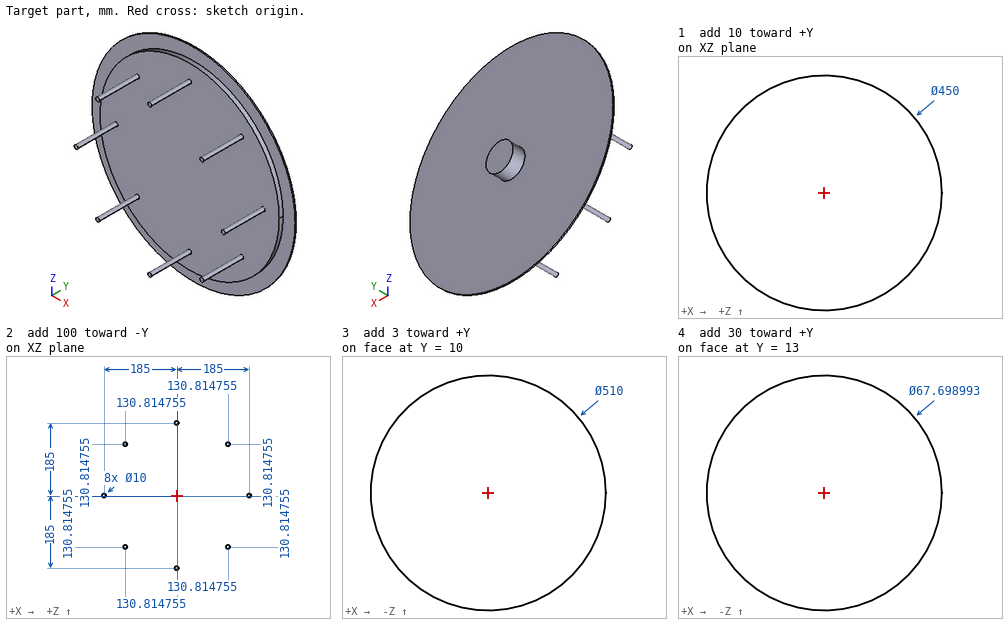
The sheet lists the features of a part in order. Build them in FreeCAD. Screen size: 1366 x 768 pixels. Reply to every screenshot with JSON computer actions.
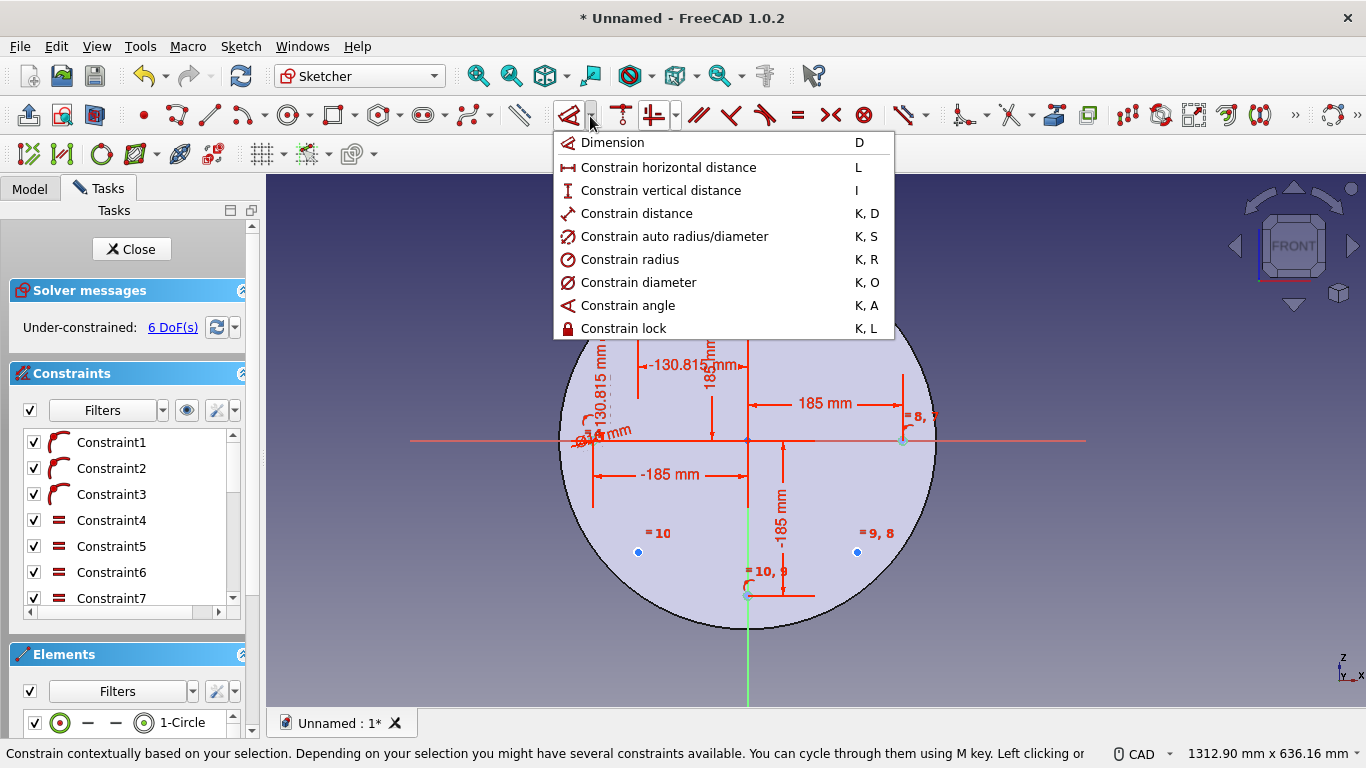
{"action": "left_click", "coordinate": [724, 168]}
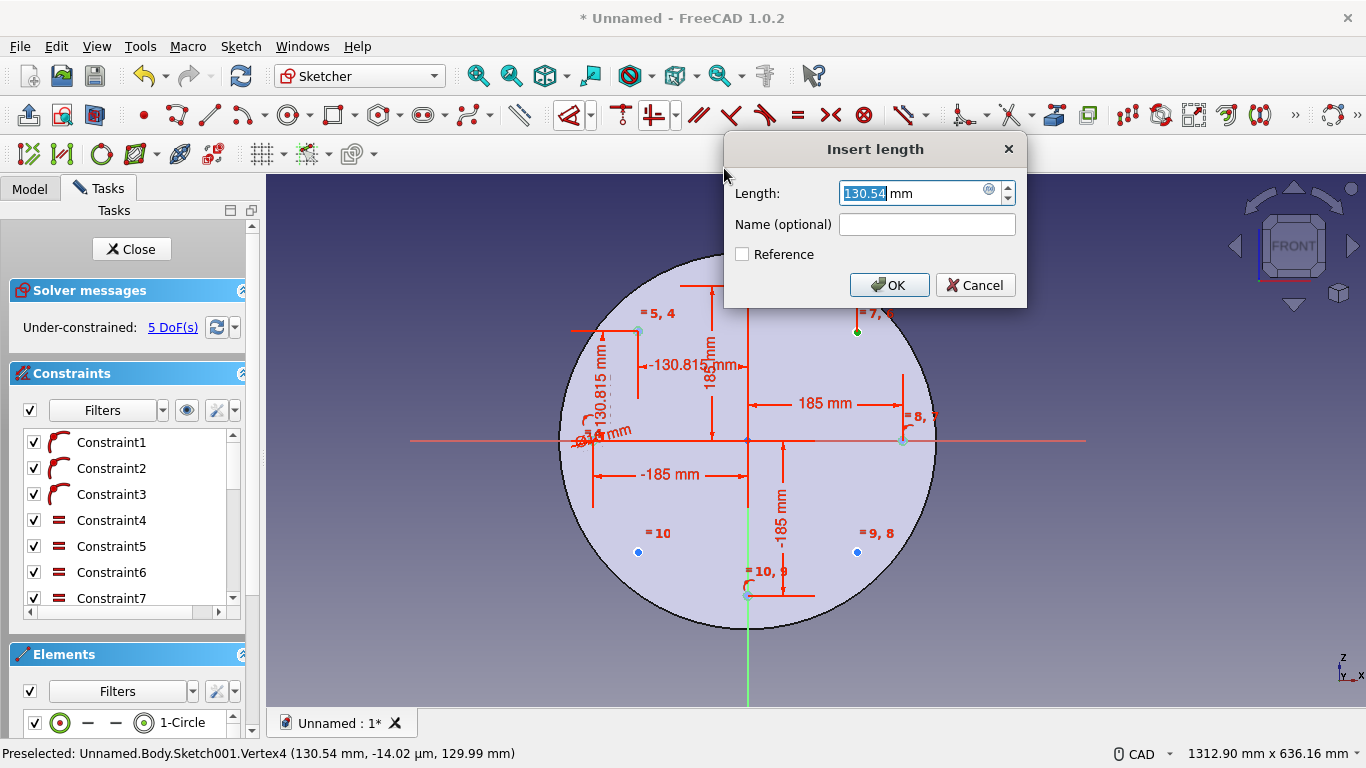
{"action": "type", "text": "130.814755"}
{"action": "key", "text": "Return"}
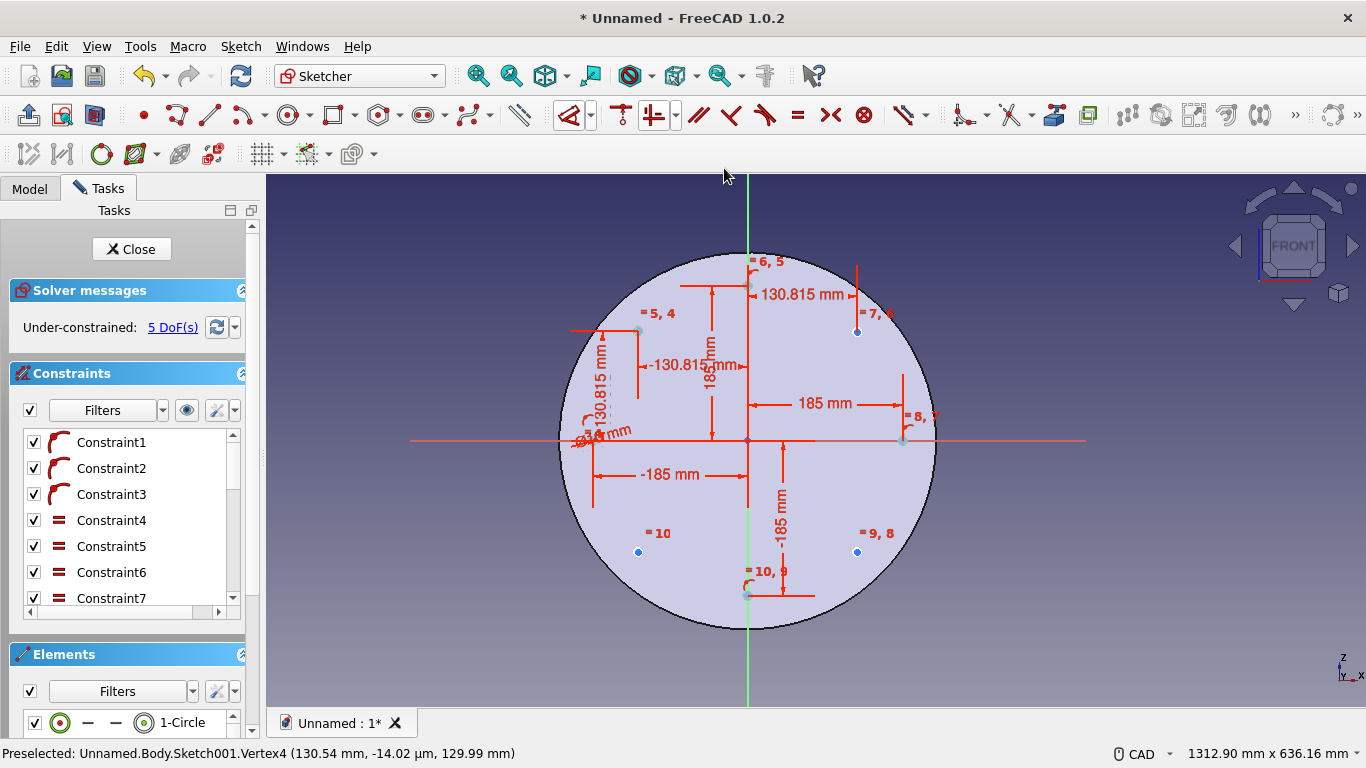
{"action": "left_click", "coordinate": [857, 332]}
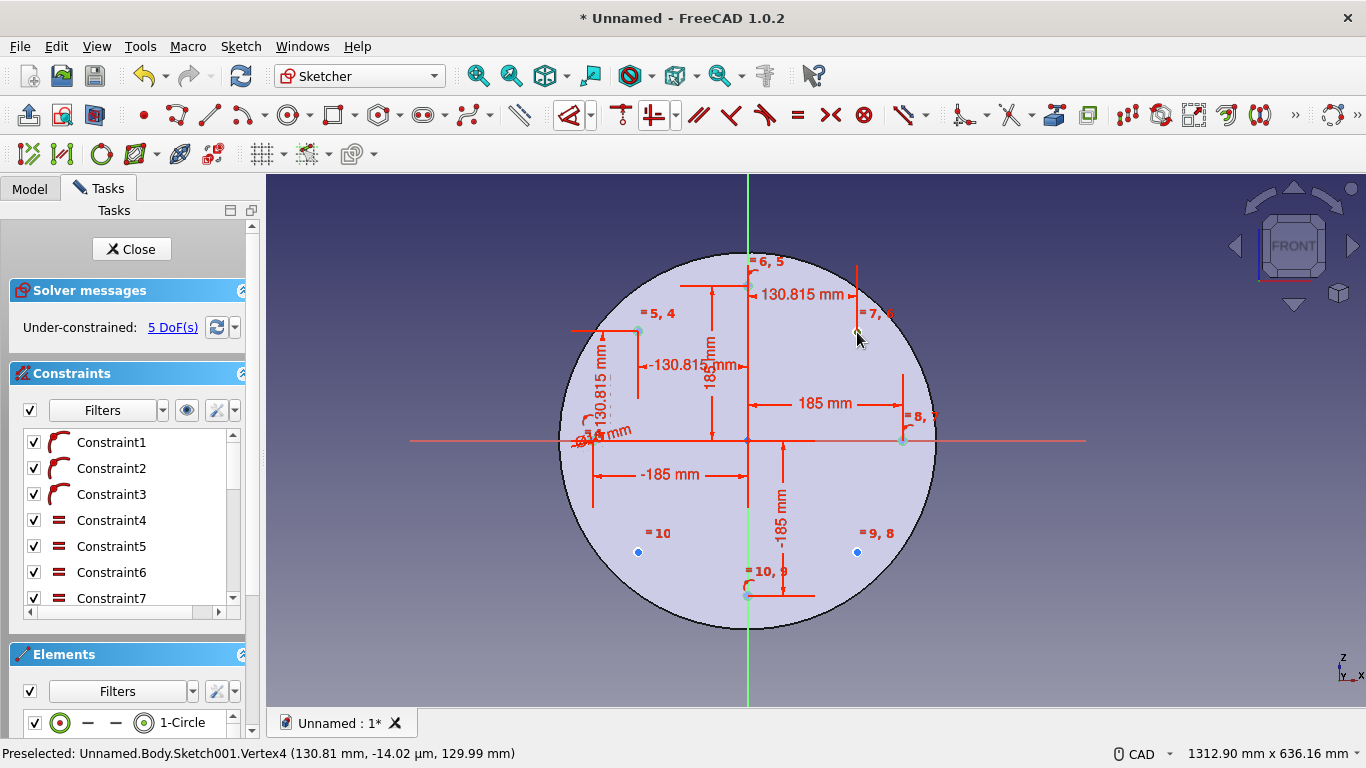
{"action": "left_click", "coordinate": [590, 116]}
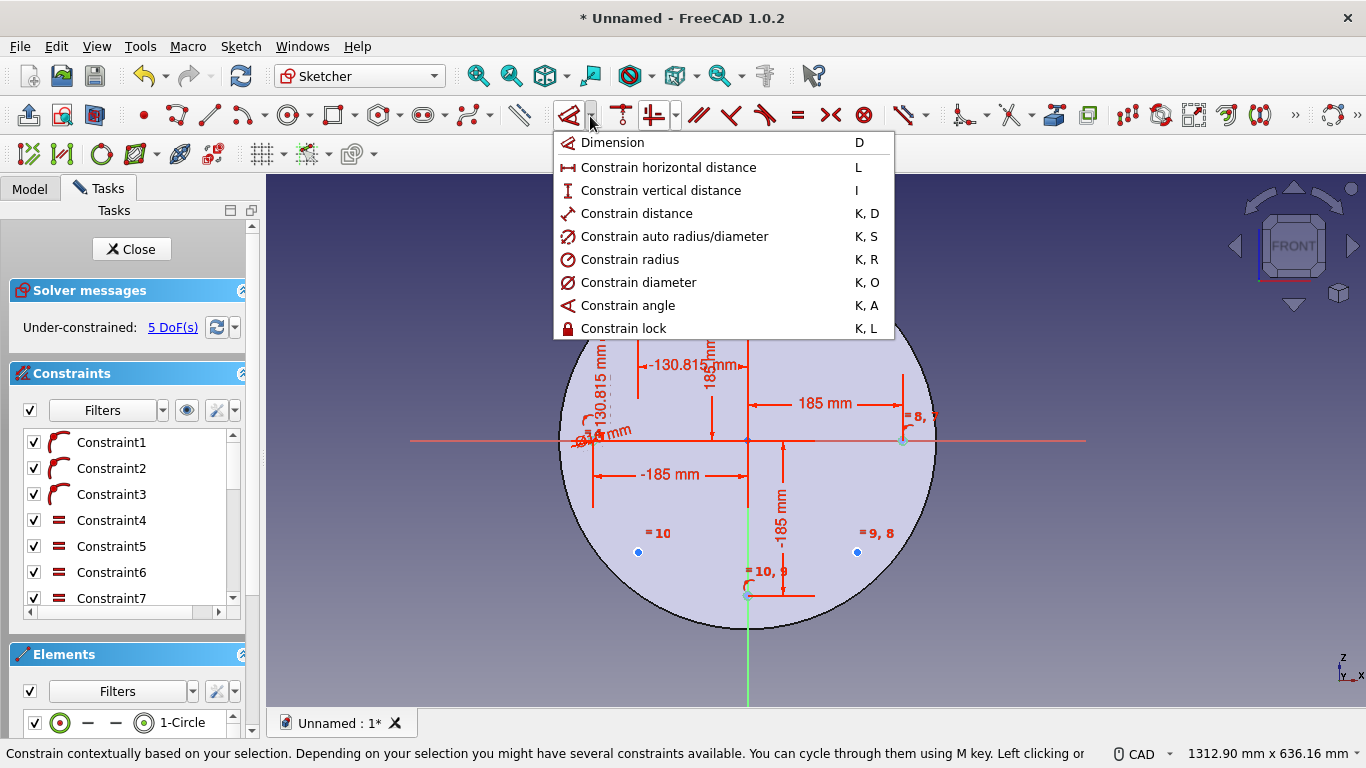
{"action": "left_click", "coordinate": [724, 190]}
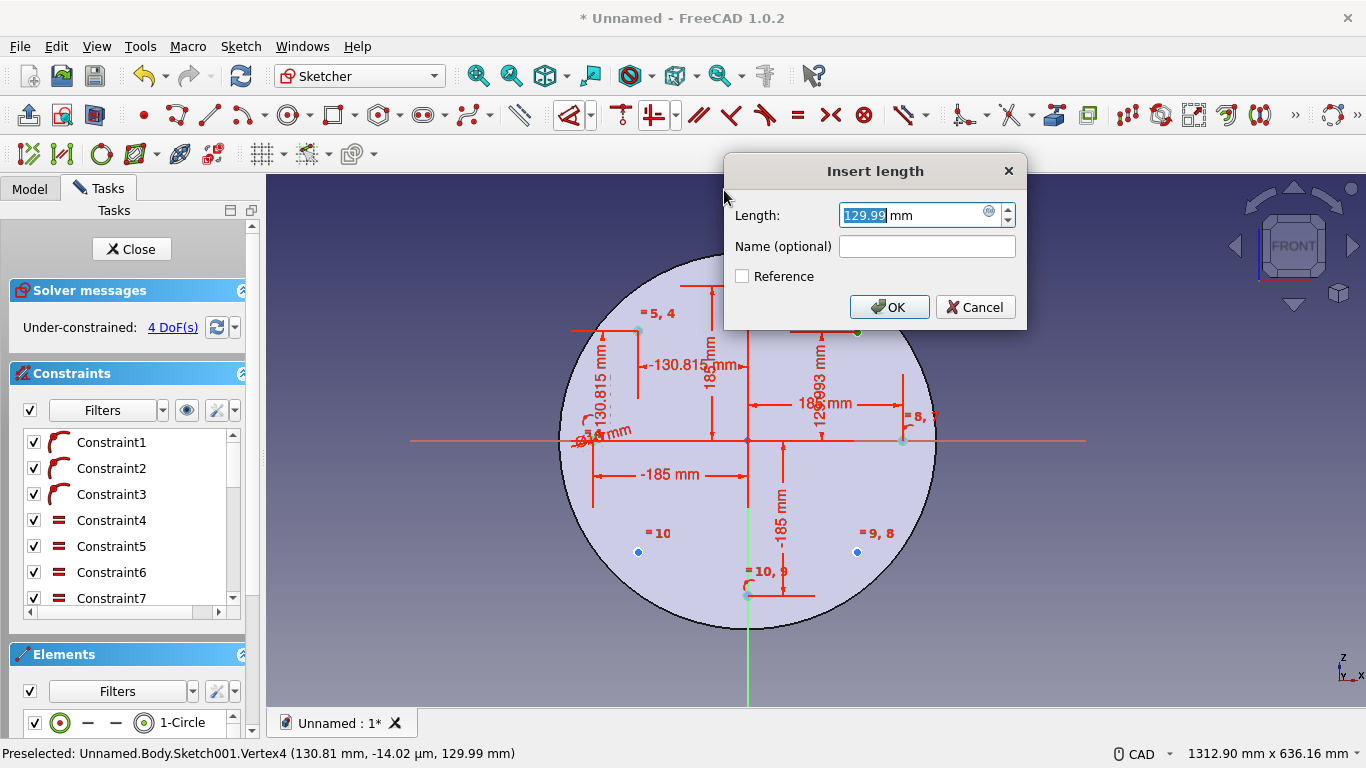
{"action": "type", "text": "130.814755"}
{"action": "key", "text": "Return"}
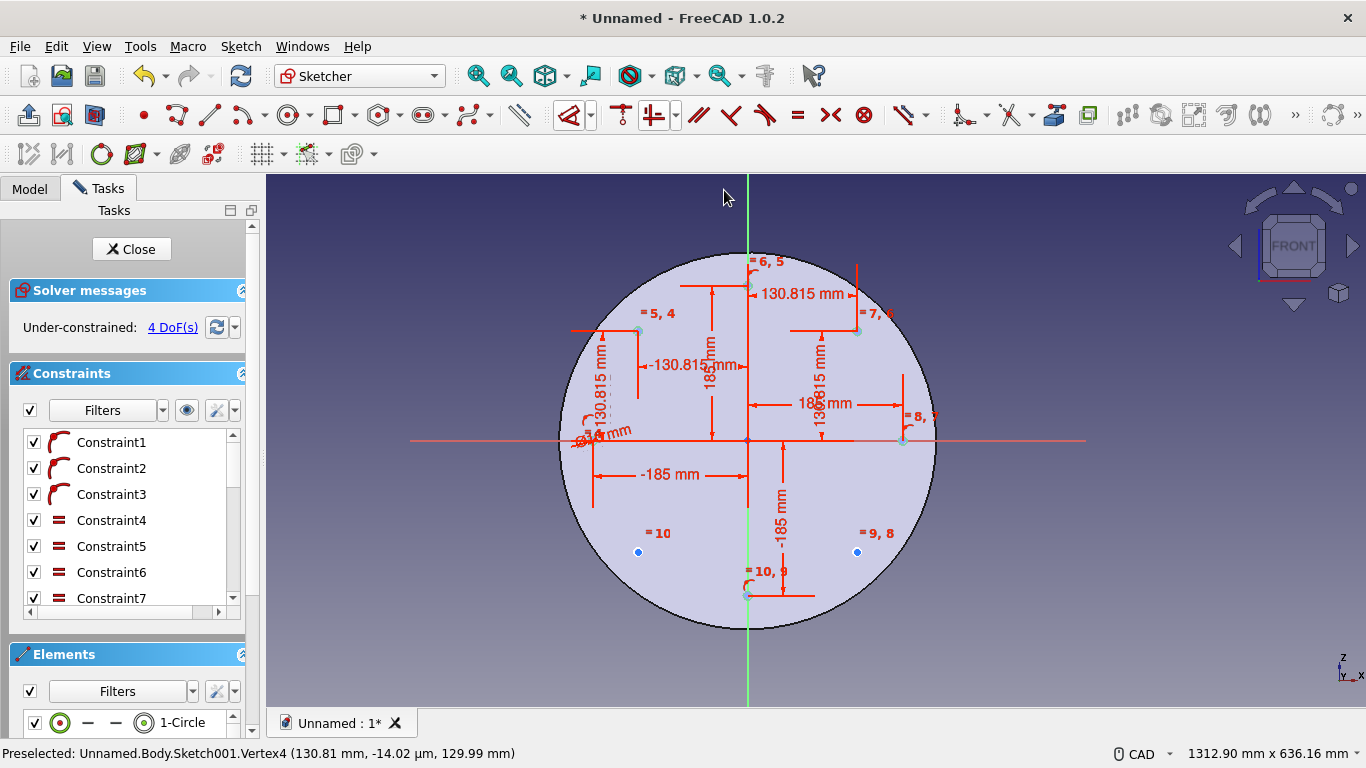
{"action": "left_click", "coordinate": [857, 552]}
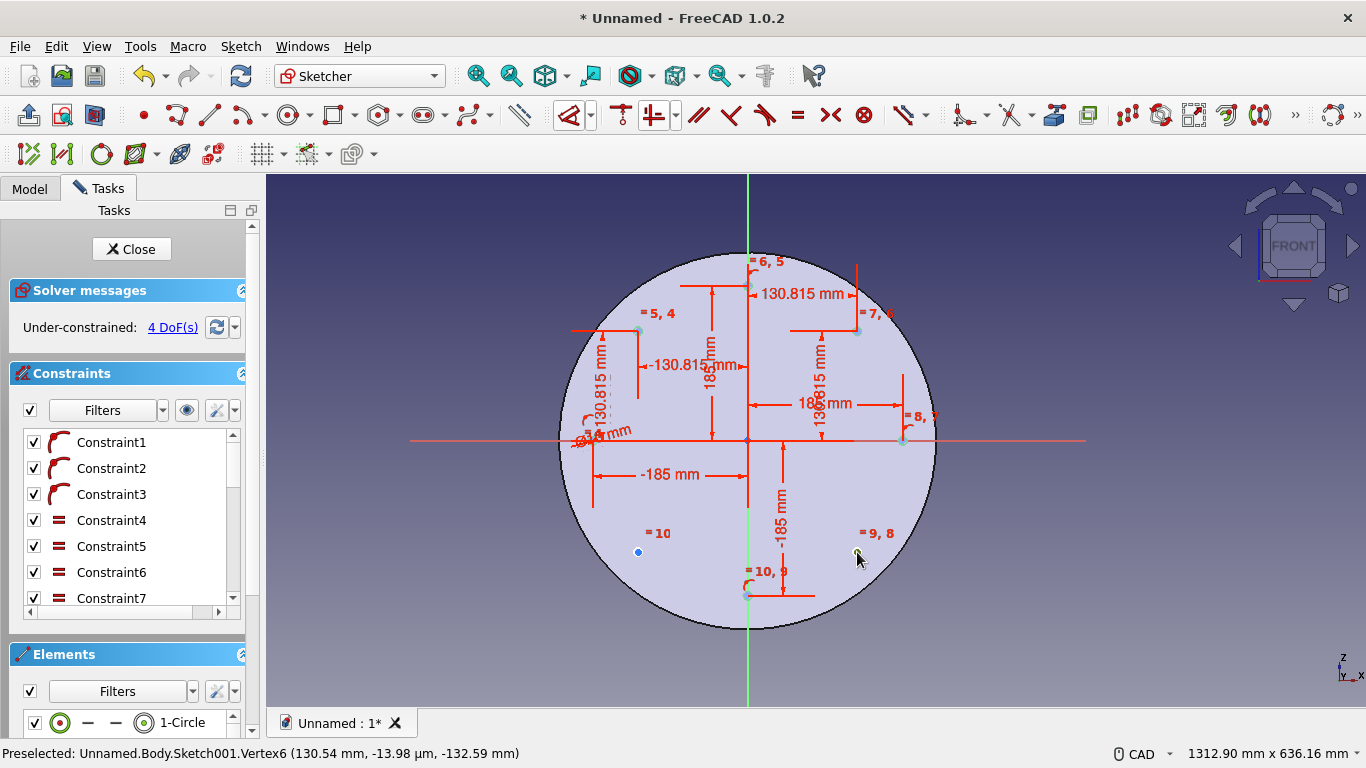
{"action": "left_click", "coordinate": [590, 116]}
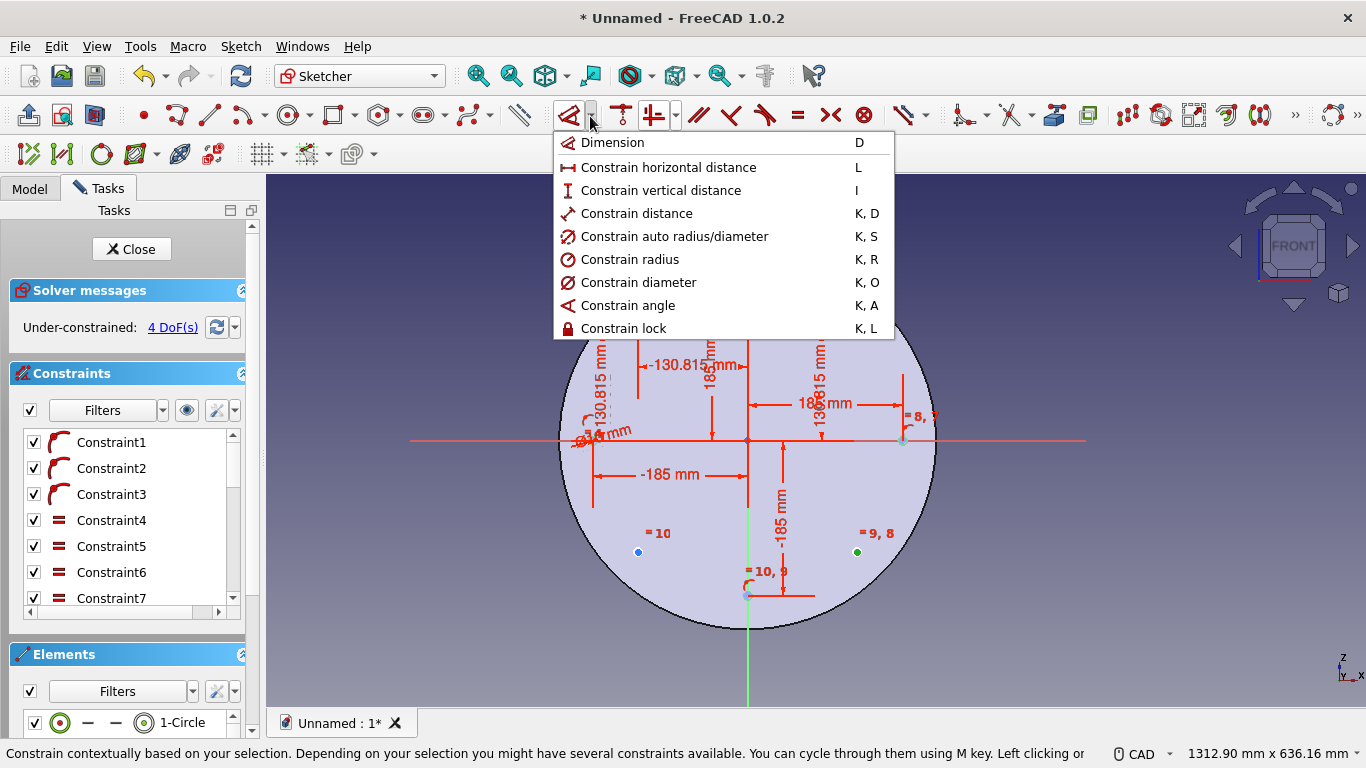
{"action": "left_click", "coordinate": [724, 168]}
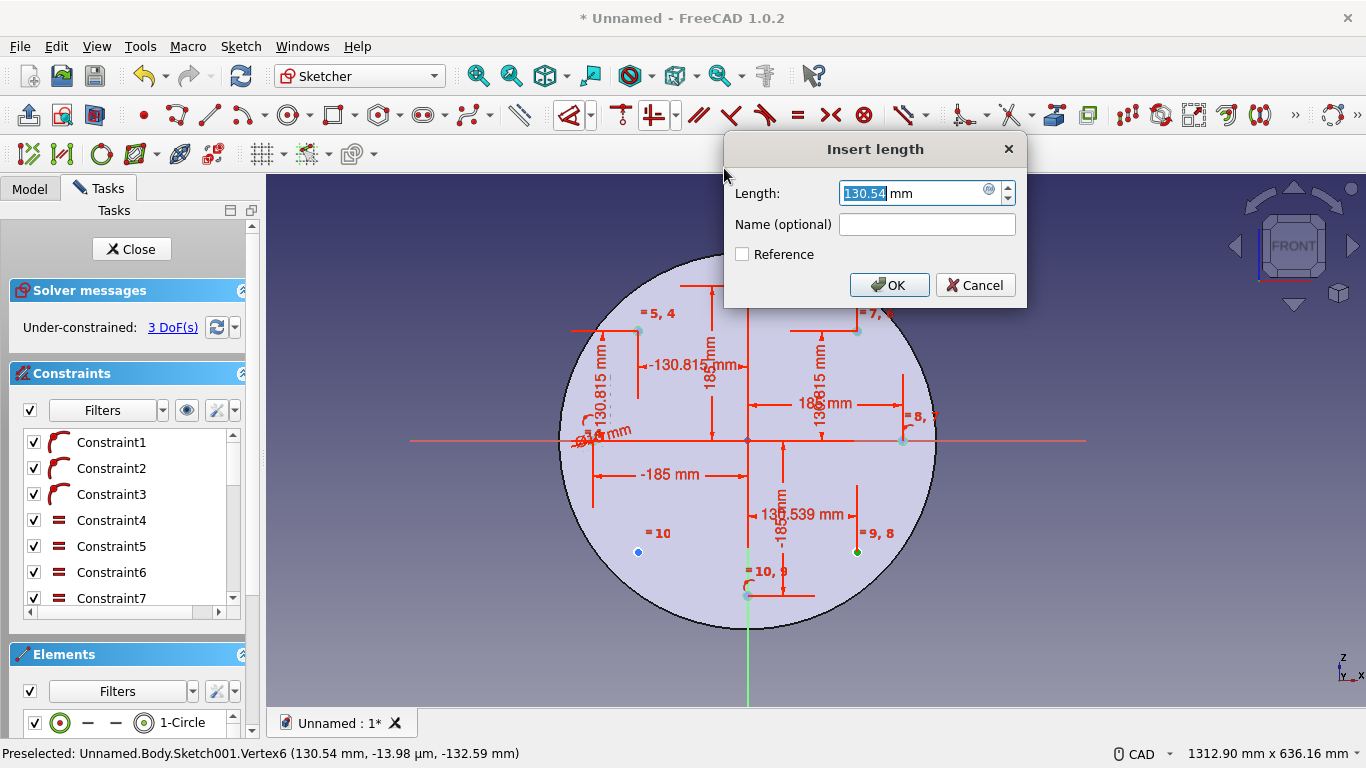
{"action": "type", "text": "130.814755"}
{"action": "key", "text": "Return"}